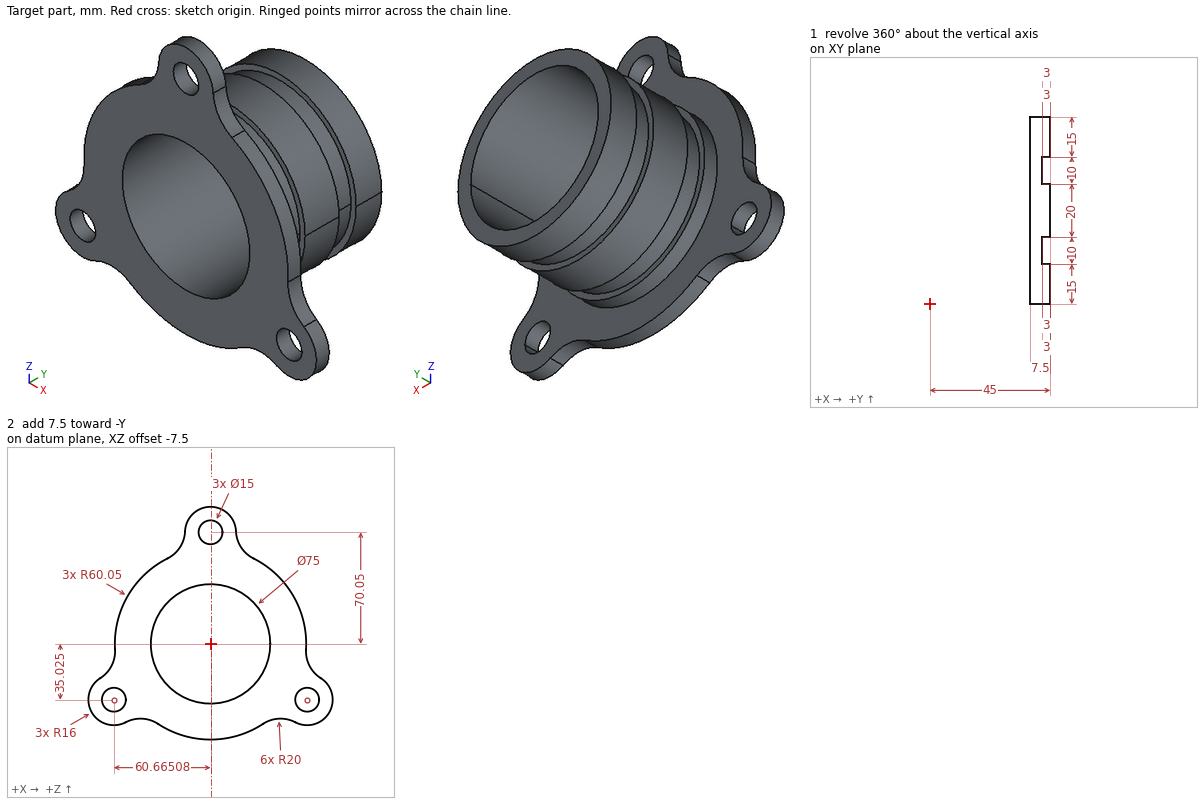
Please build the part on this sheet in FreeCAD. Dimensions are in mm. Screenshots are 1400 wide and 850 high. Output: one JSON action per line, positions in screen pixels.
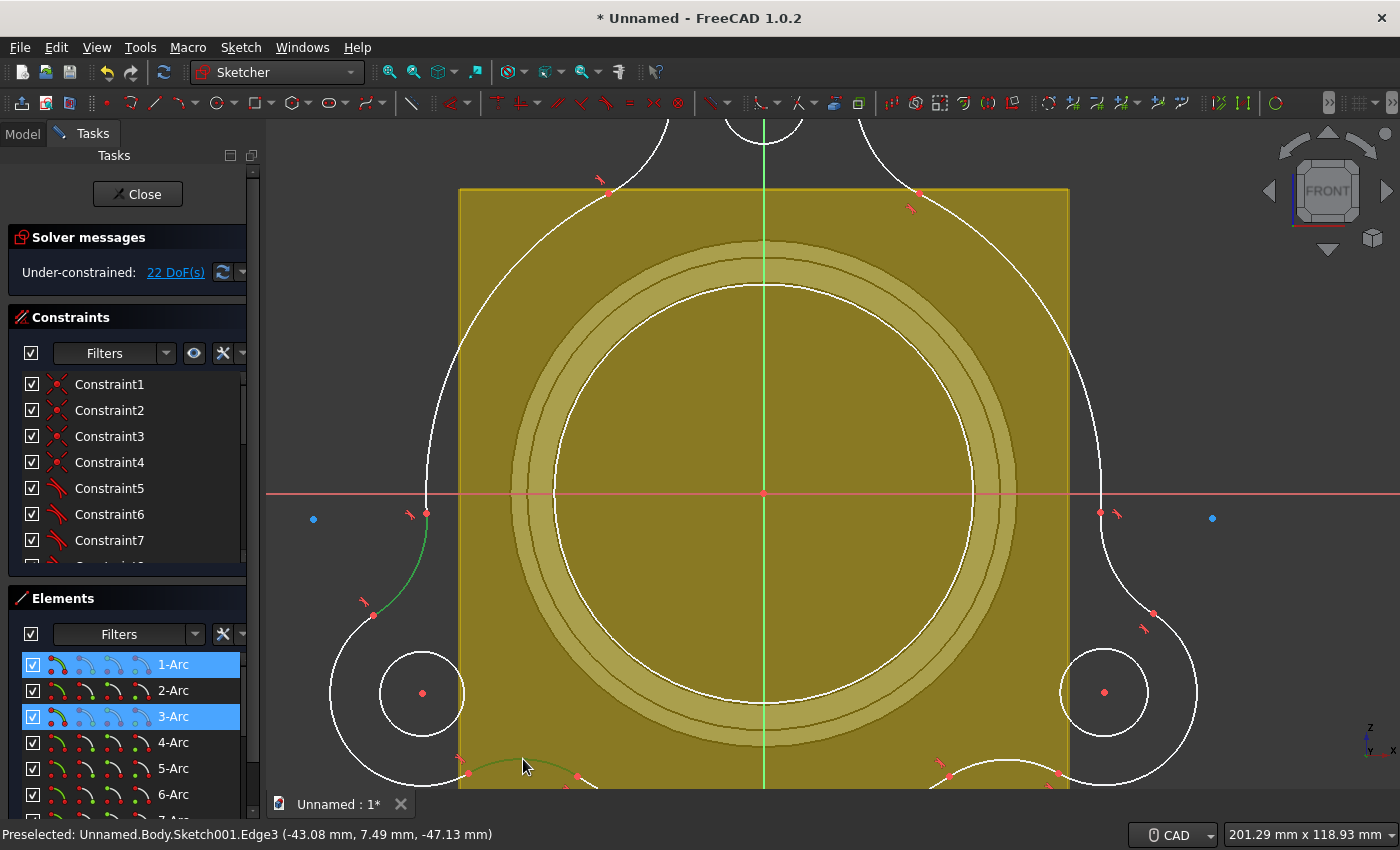
{"action": "left_click", "coordinate": [1003, 760]}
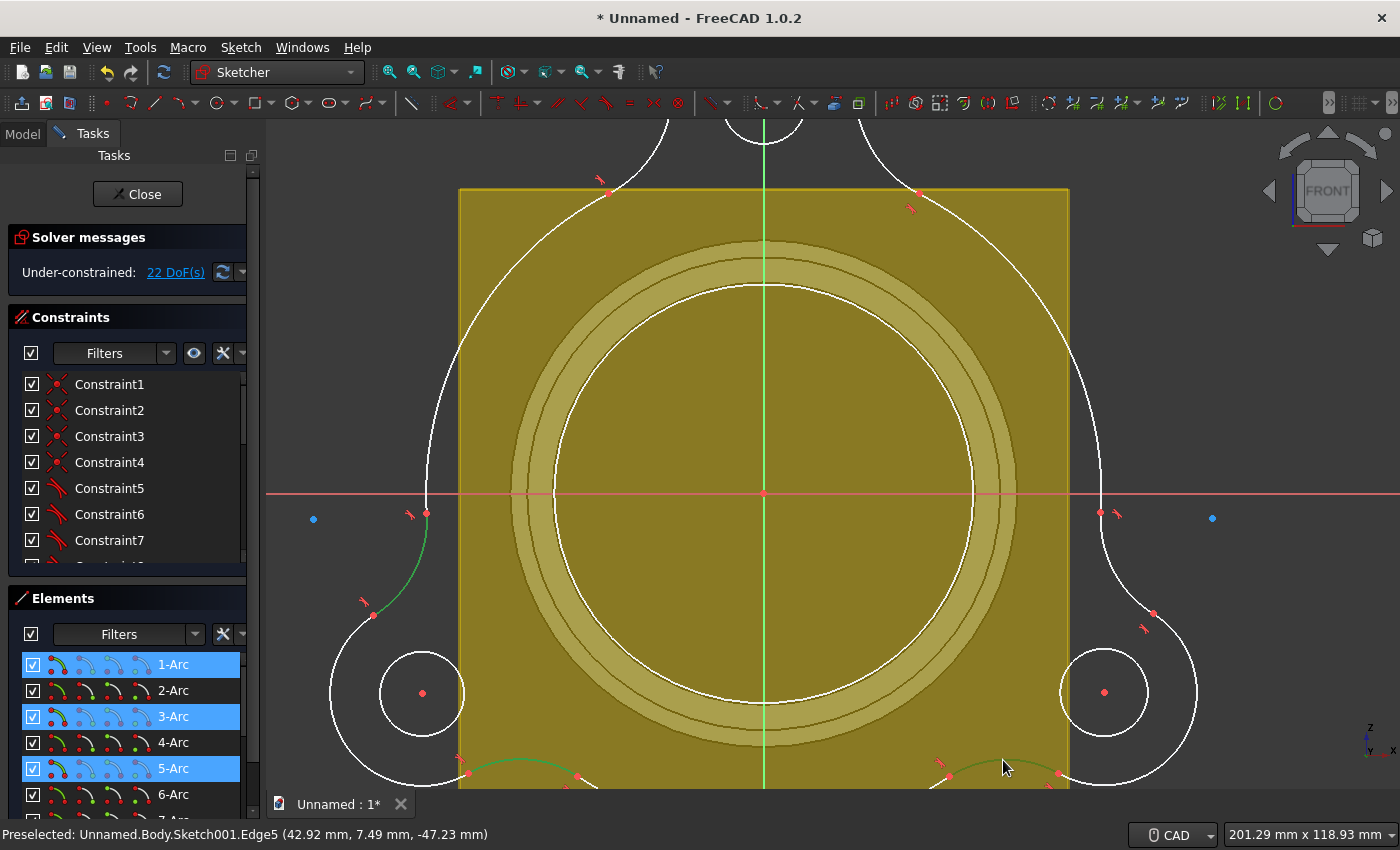
{"action": "left_click", "coordinate": [1105, 548]}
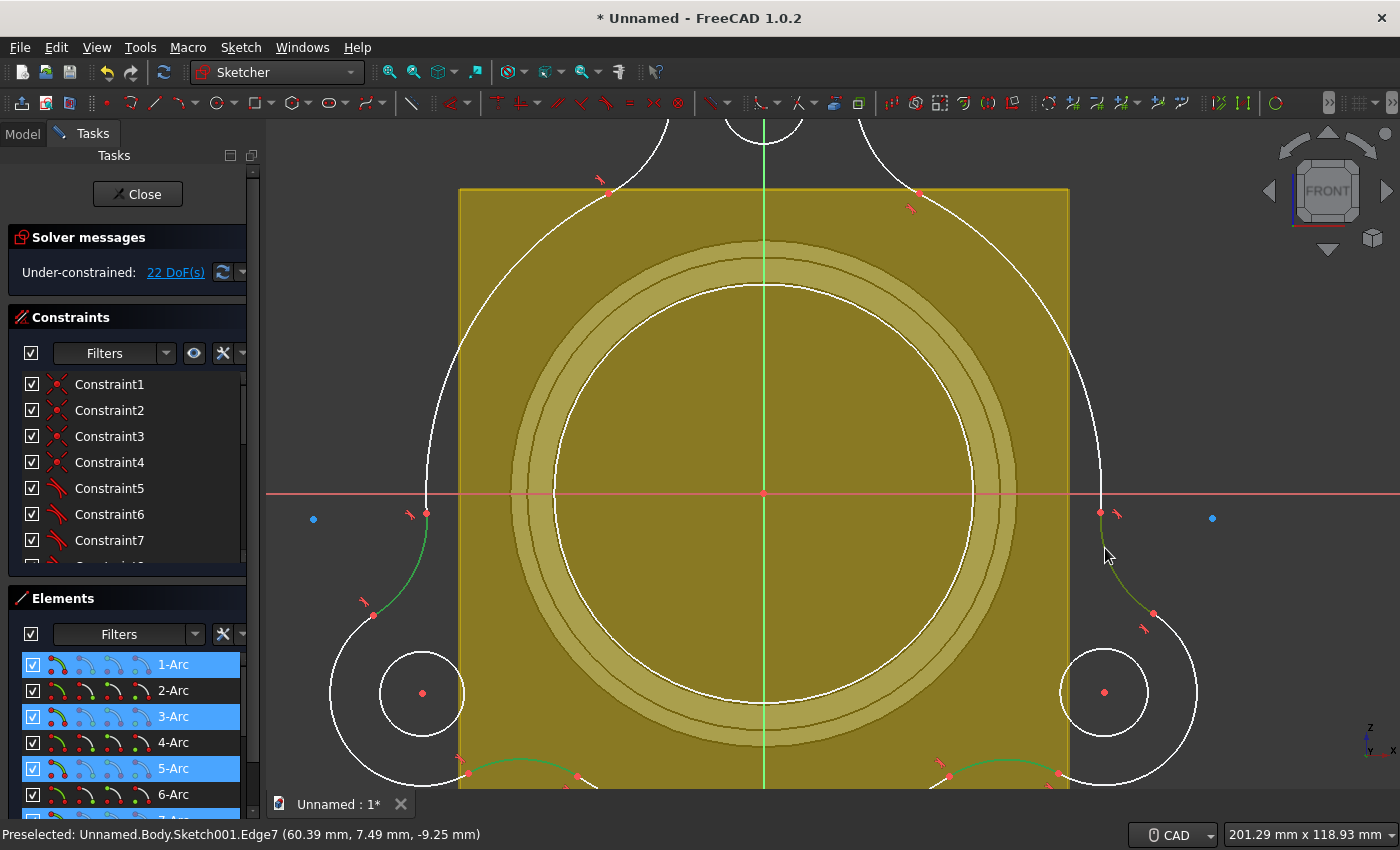
{"action": "left_click", "coordinate": [890, 172]}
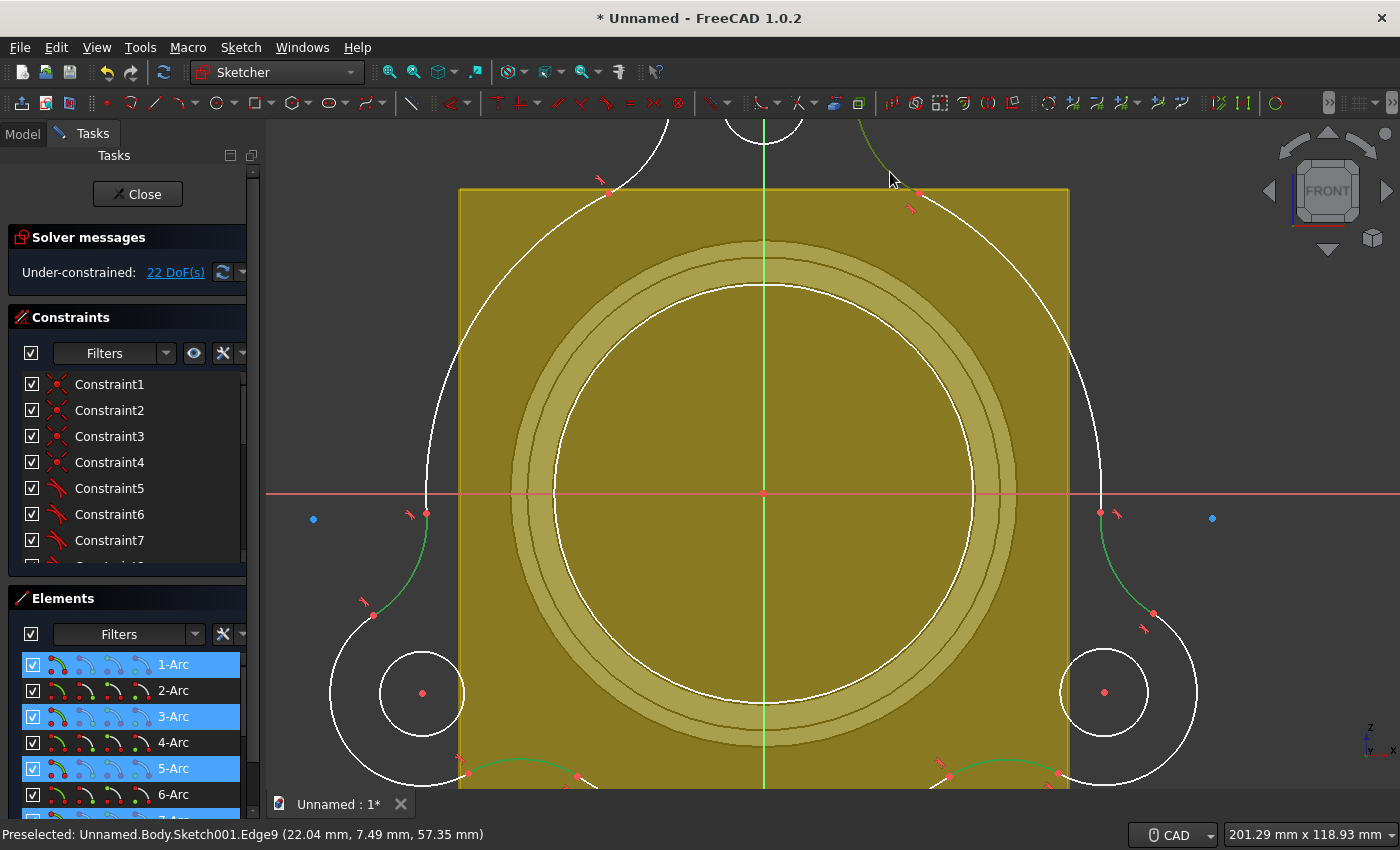
{"action": "left_click", "coordinate": [638, 172]}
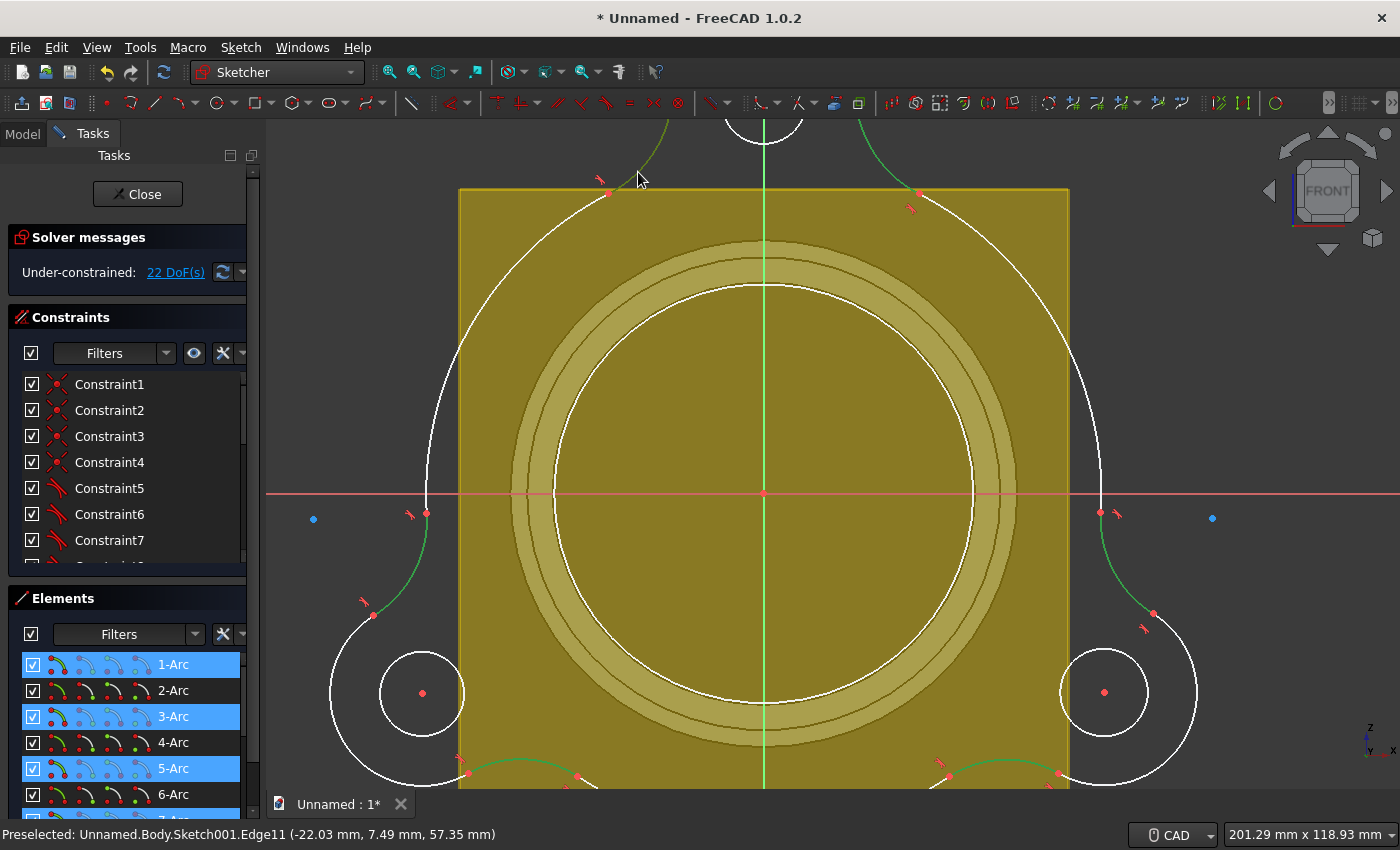
{"action": "left_click", "coordinate": [630, 104]}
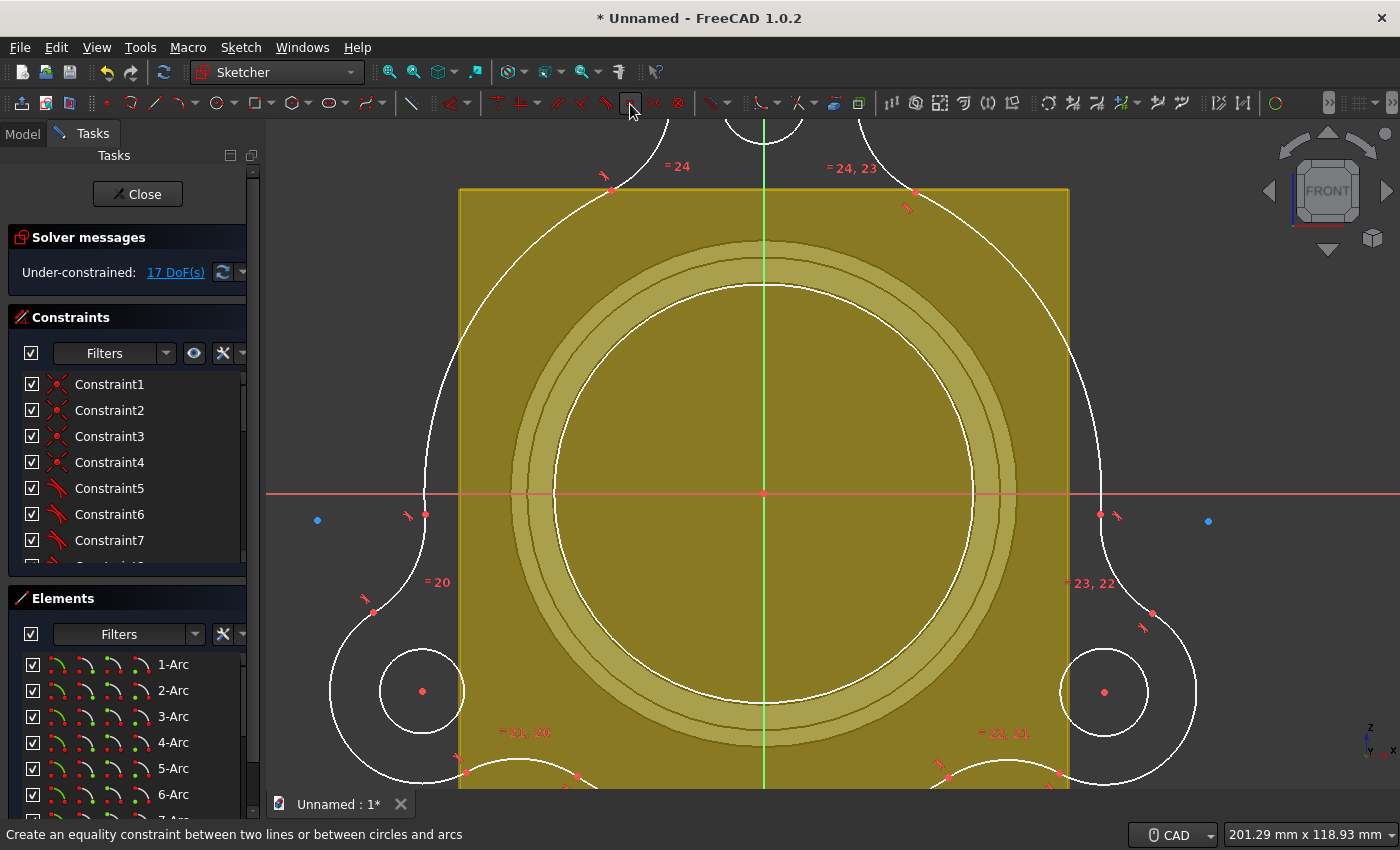
{"action": "left_click", "coordinate": [330, 683]}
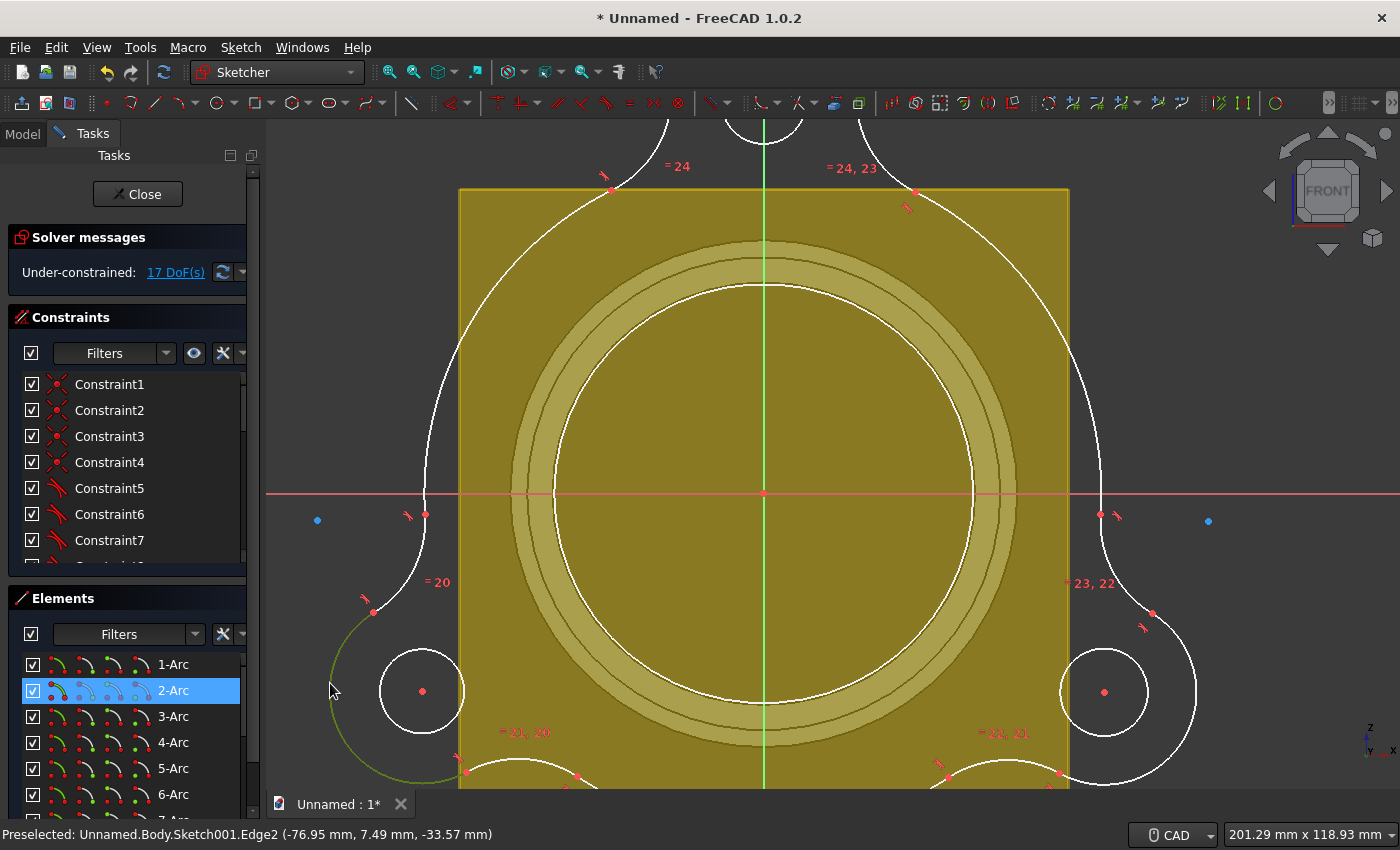
{"action": "left_click", "coordinate": [1196, 684]}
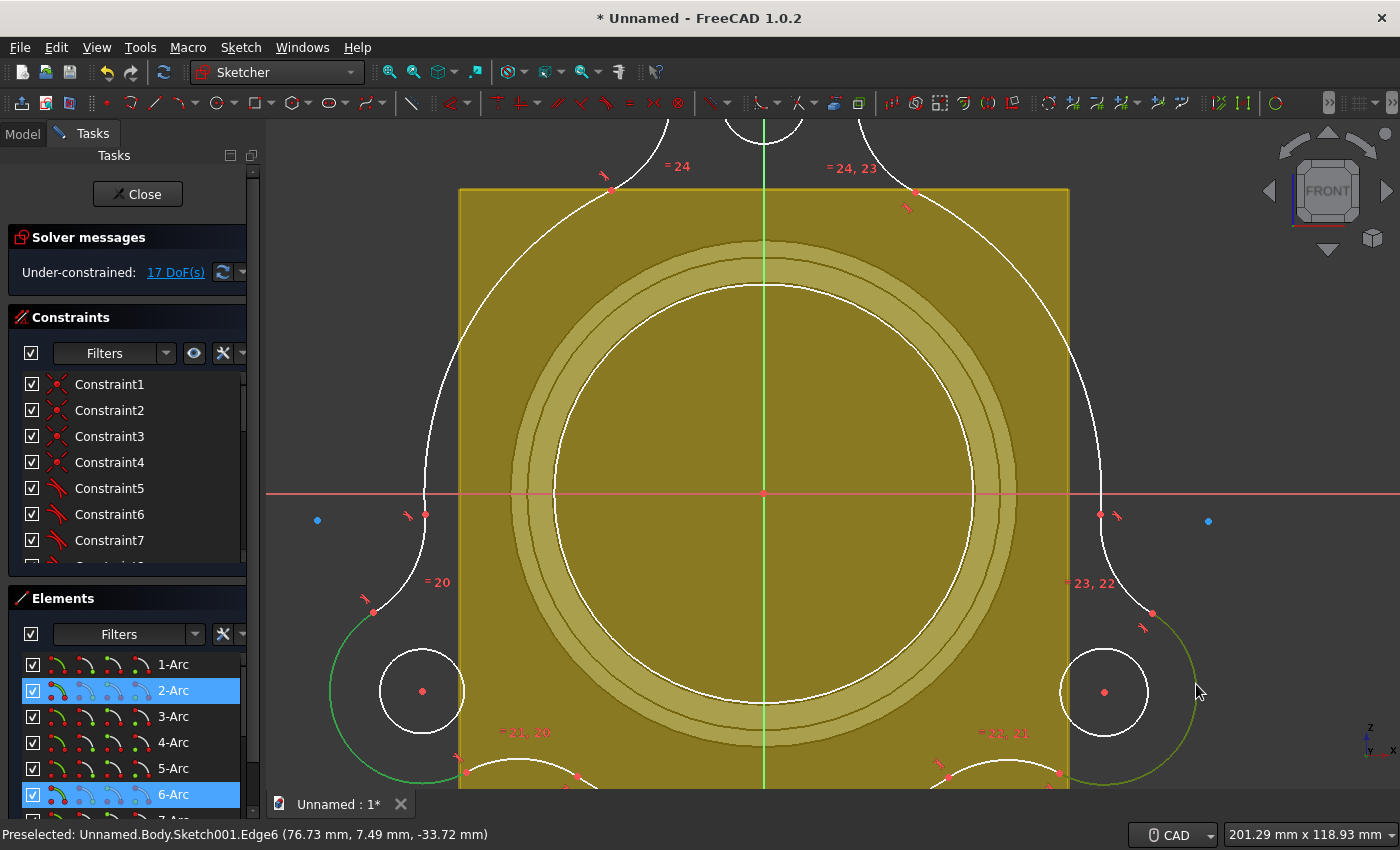
{"action": "scroll", "coordinate": [765, 495], "scroll_direction": "down", "scroll_amount": 3}